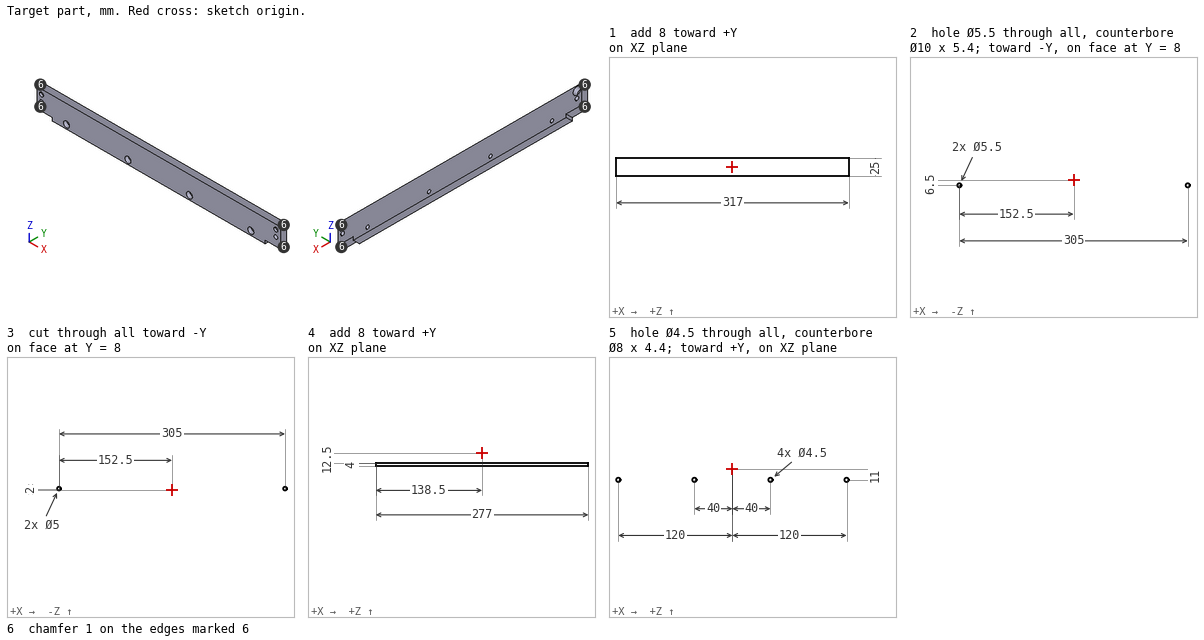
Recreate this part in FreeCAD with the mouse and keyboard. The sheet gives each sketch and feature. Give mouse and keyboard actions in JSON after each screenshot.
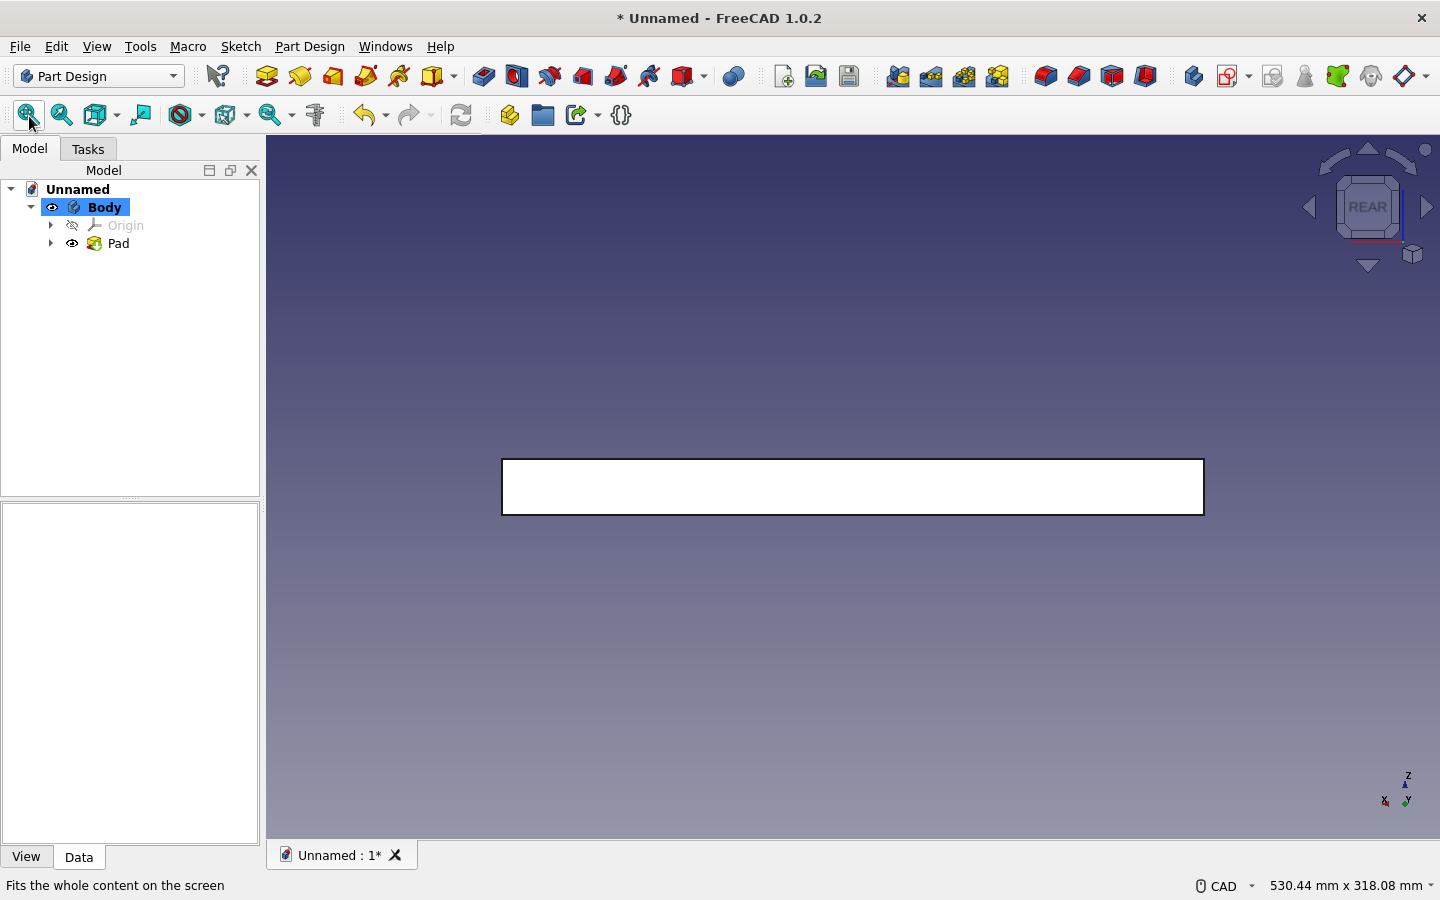
{"action": "left_click", "coordinate": [552, 486]}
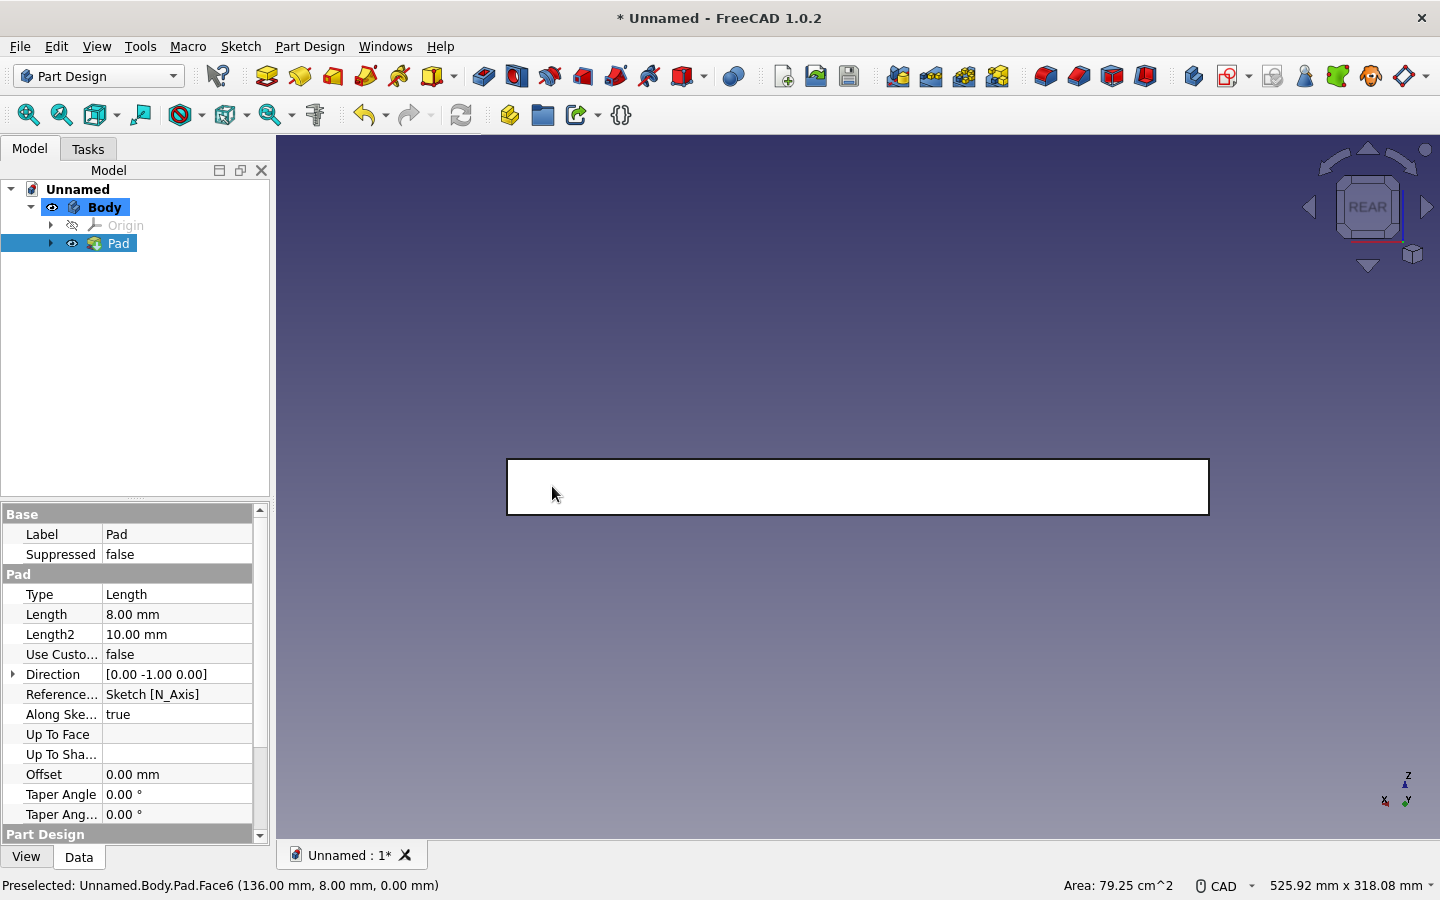
{"action": "left_click", "coordinate": [1226, 76]}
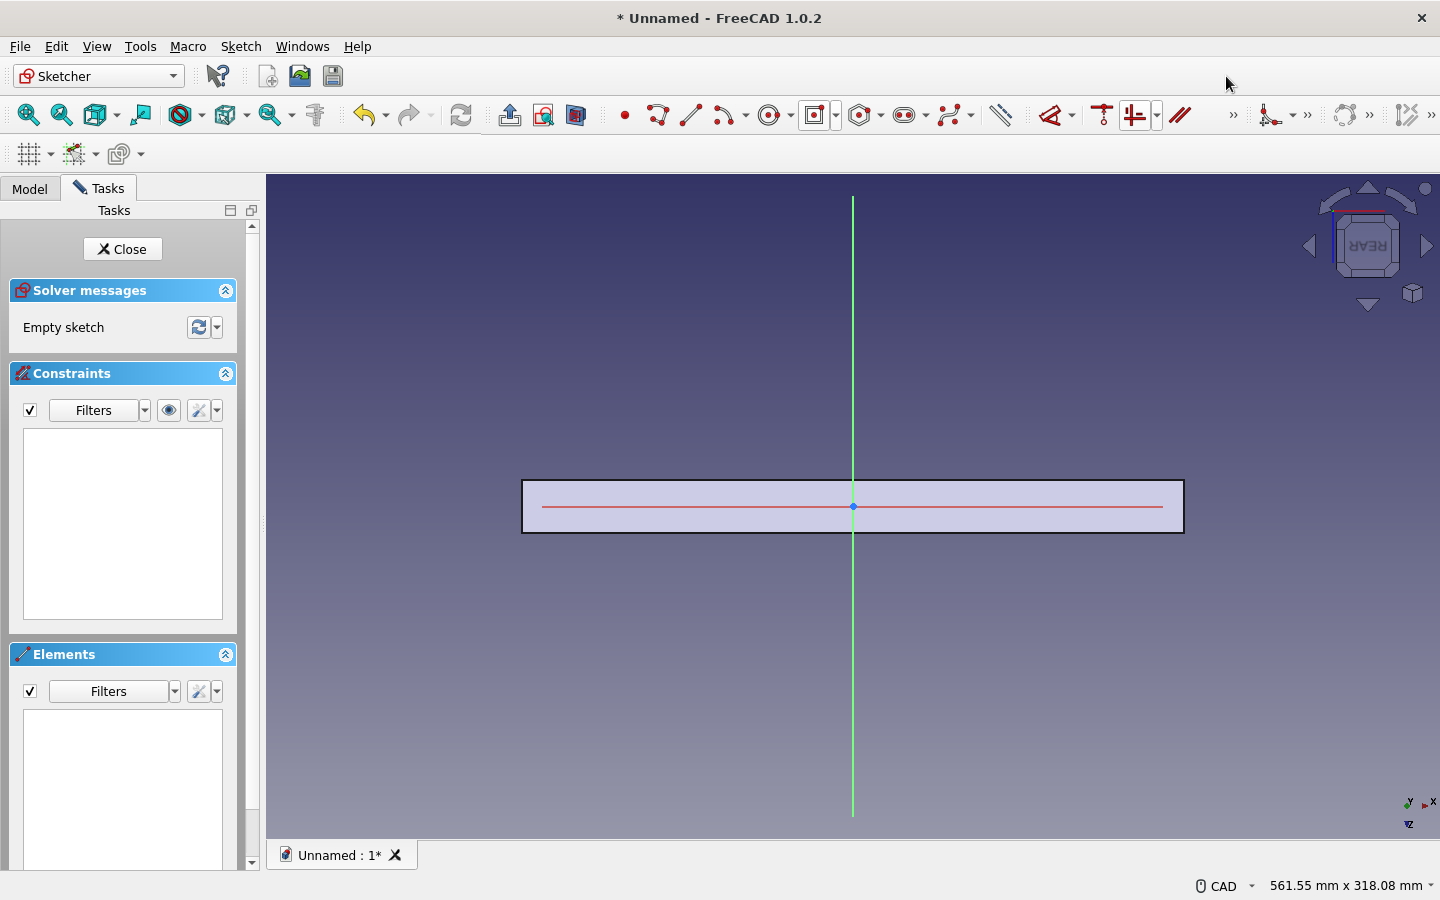
{"action": "left_click", "coordinate": [768, 116]}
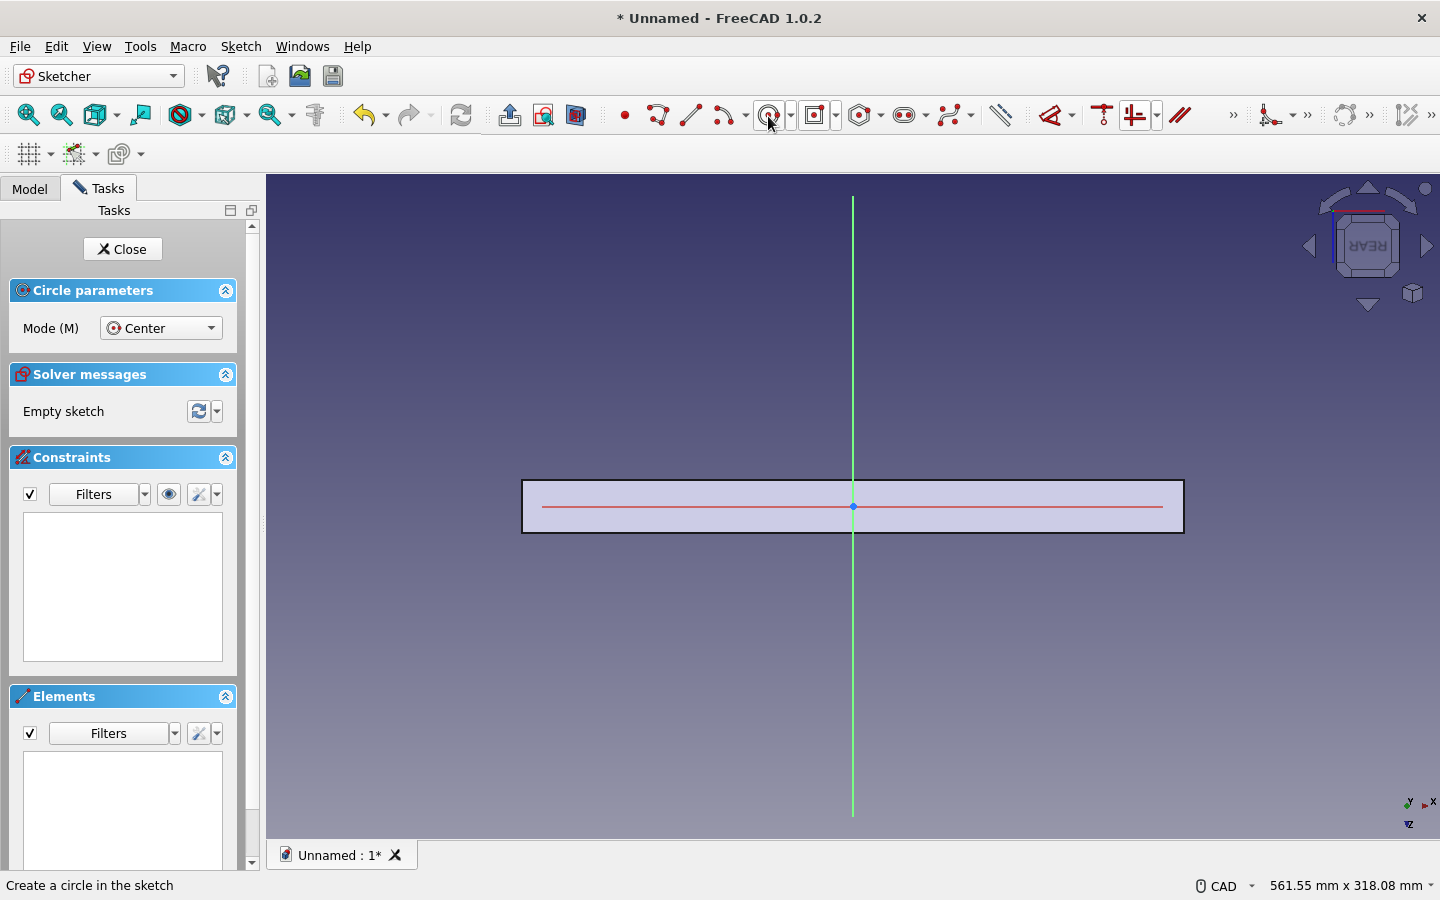
{"action": "scroll", "coordinate": [534, 520], "scroll_direction": "up", "scroll_amount": 7}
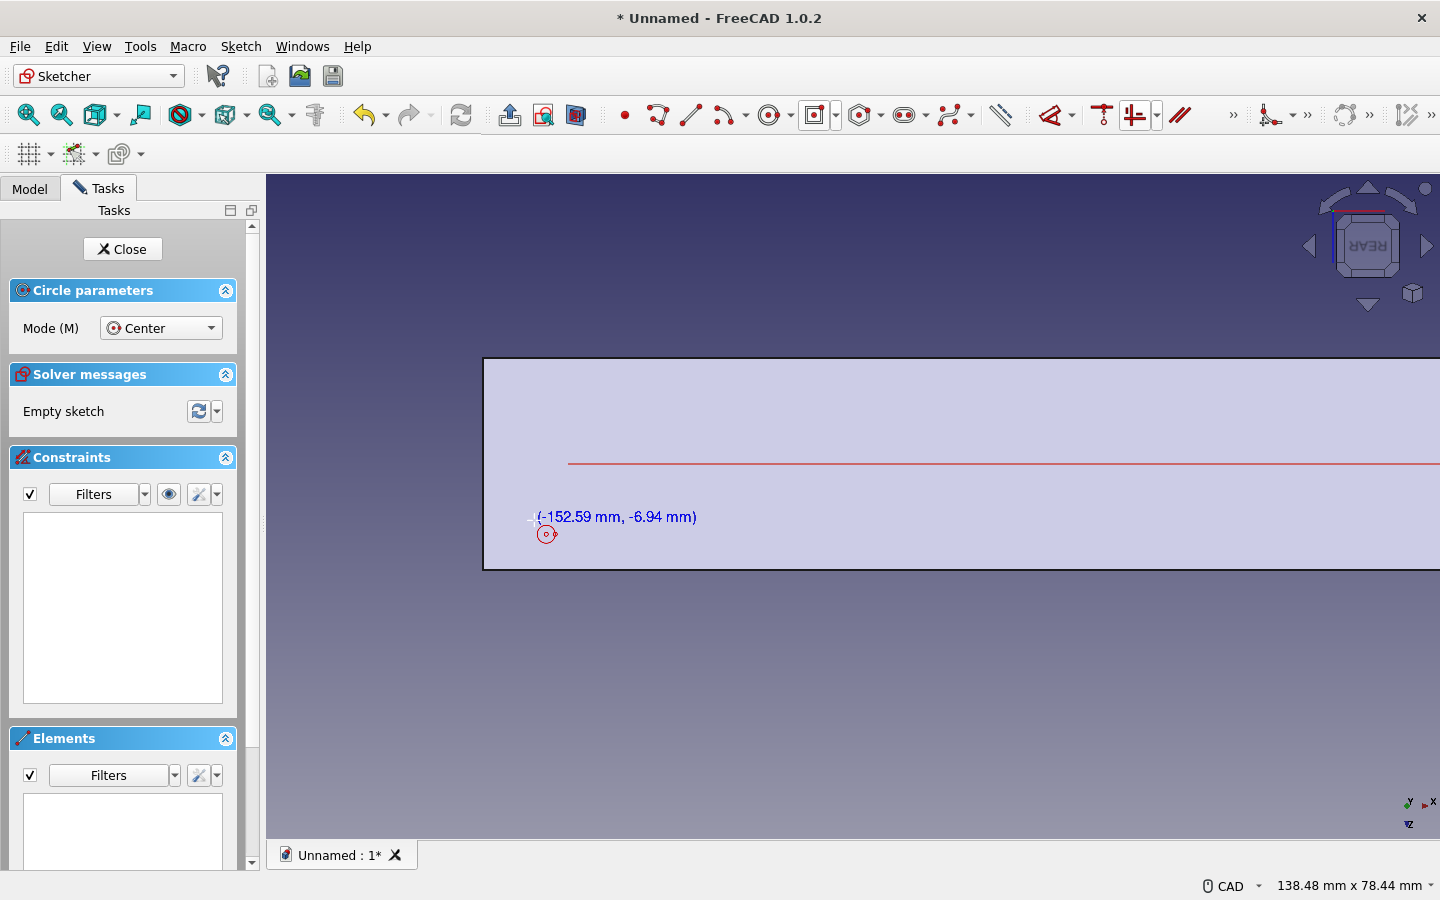
{"action": "scroll", "coordinate": [443, 508], "scroll_direction": "down", "scroll_amount": 7}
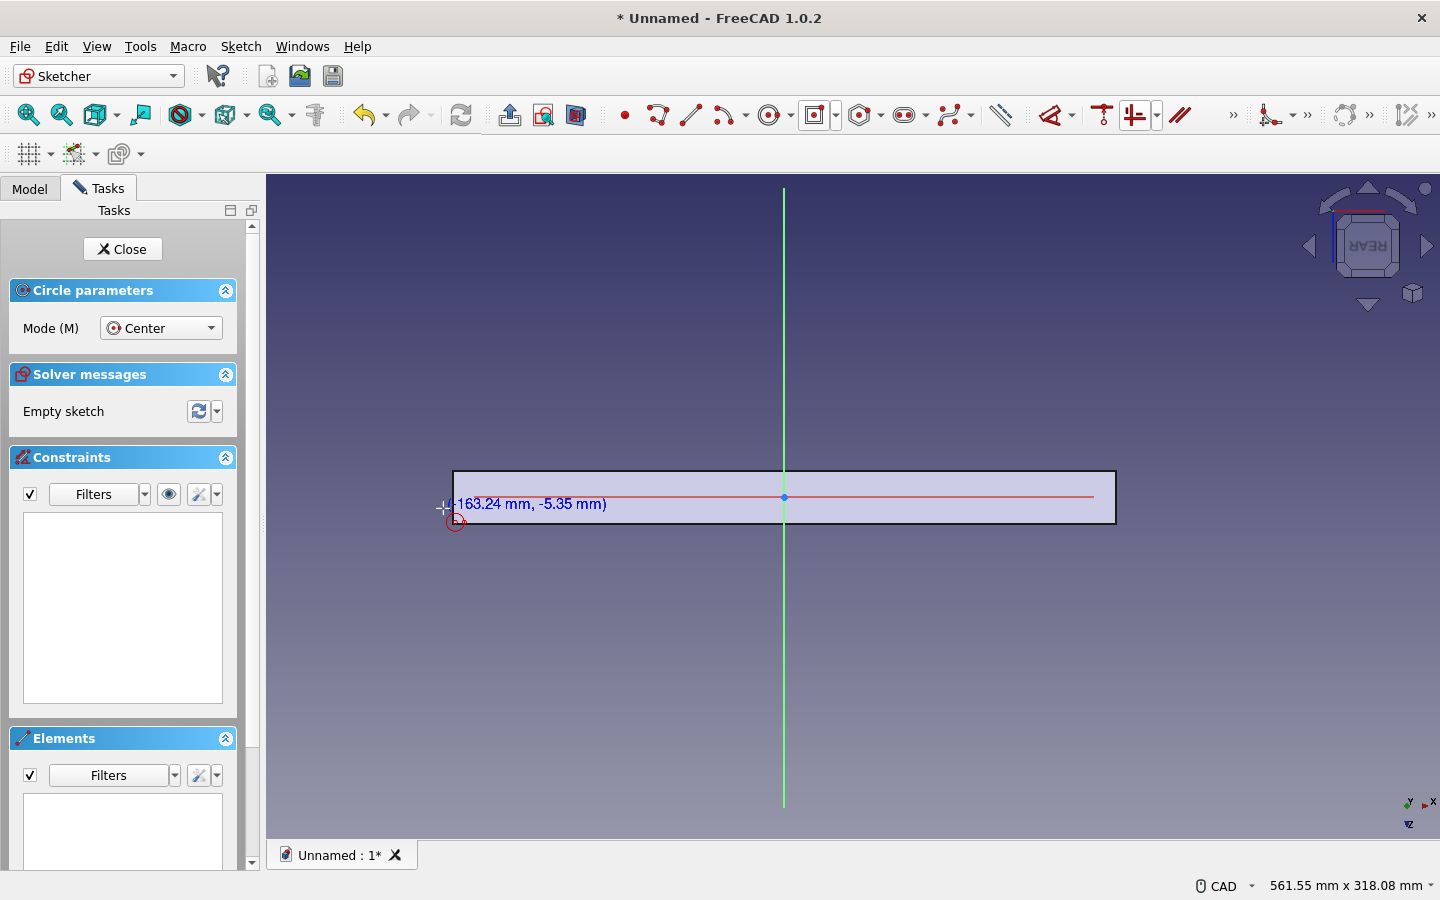
{"action": "left_click", "coordinate": [466, 511]}
{"action": "mouse_move", "coordinate": [470, 515]}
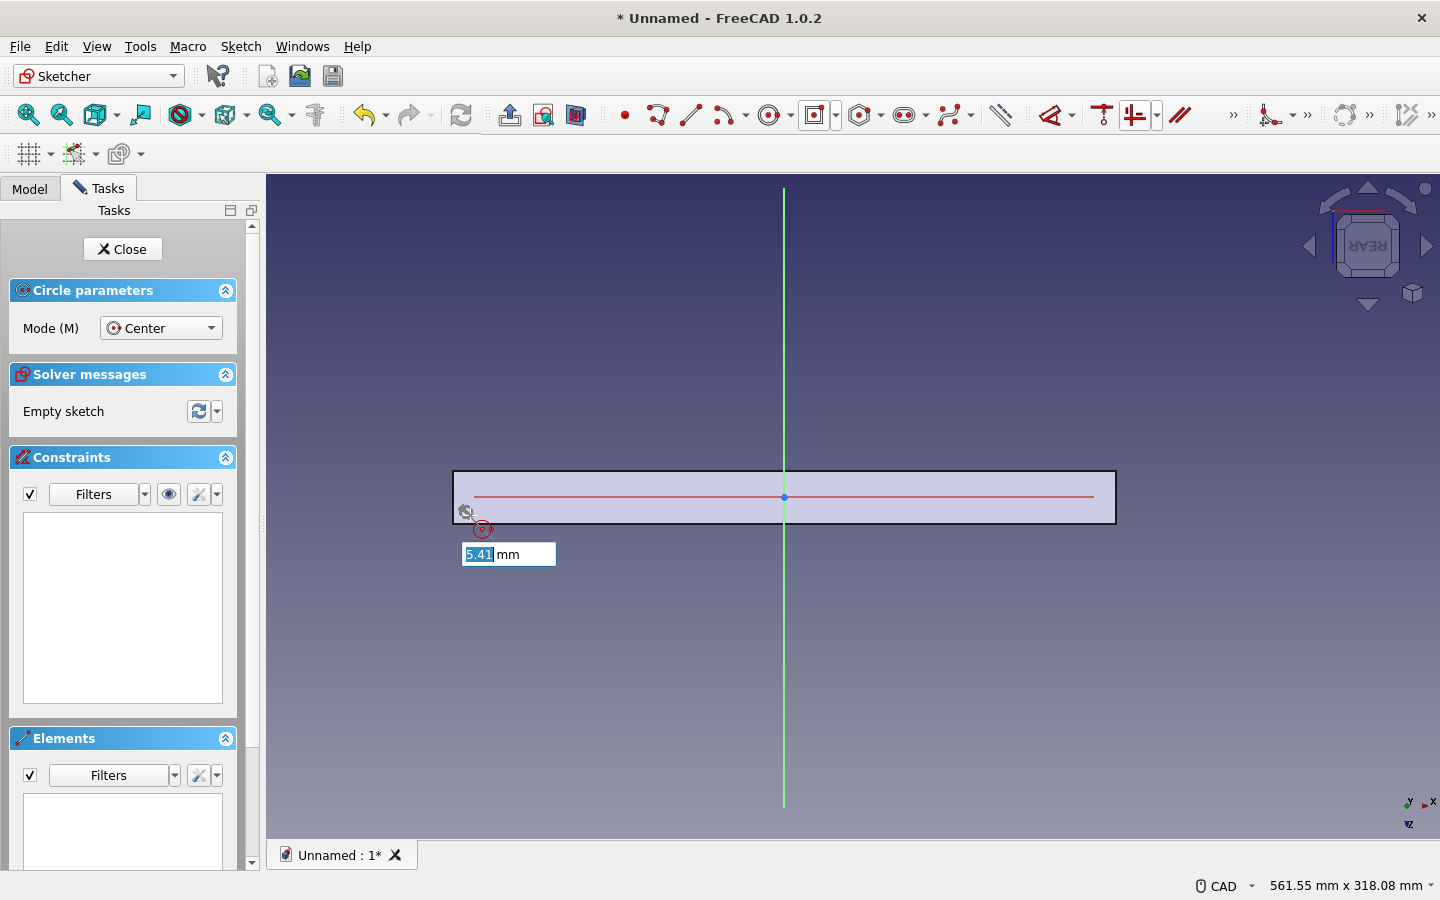
{"action": "type", "text": "5.5"}
{"action": "key", "text": "Return"}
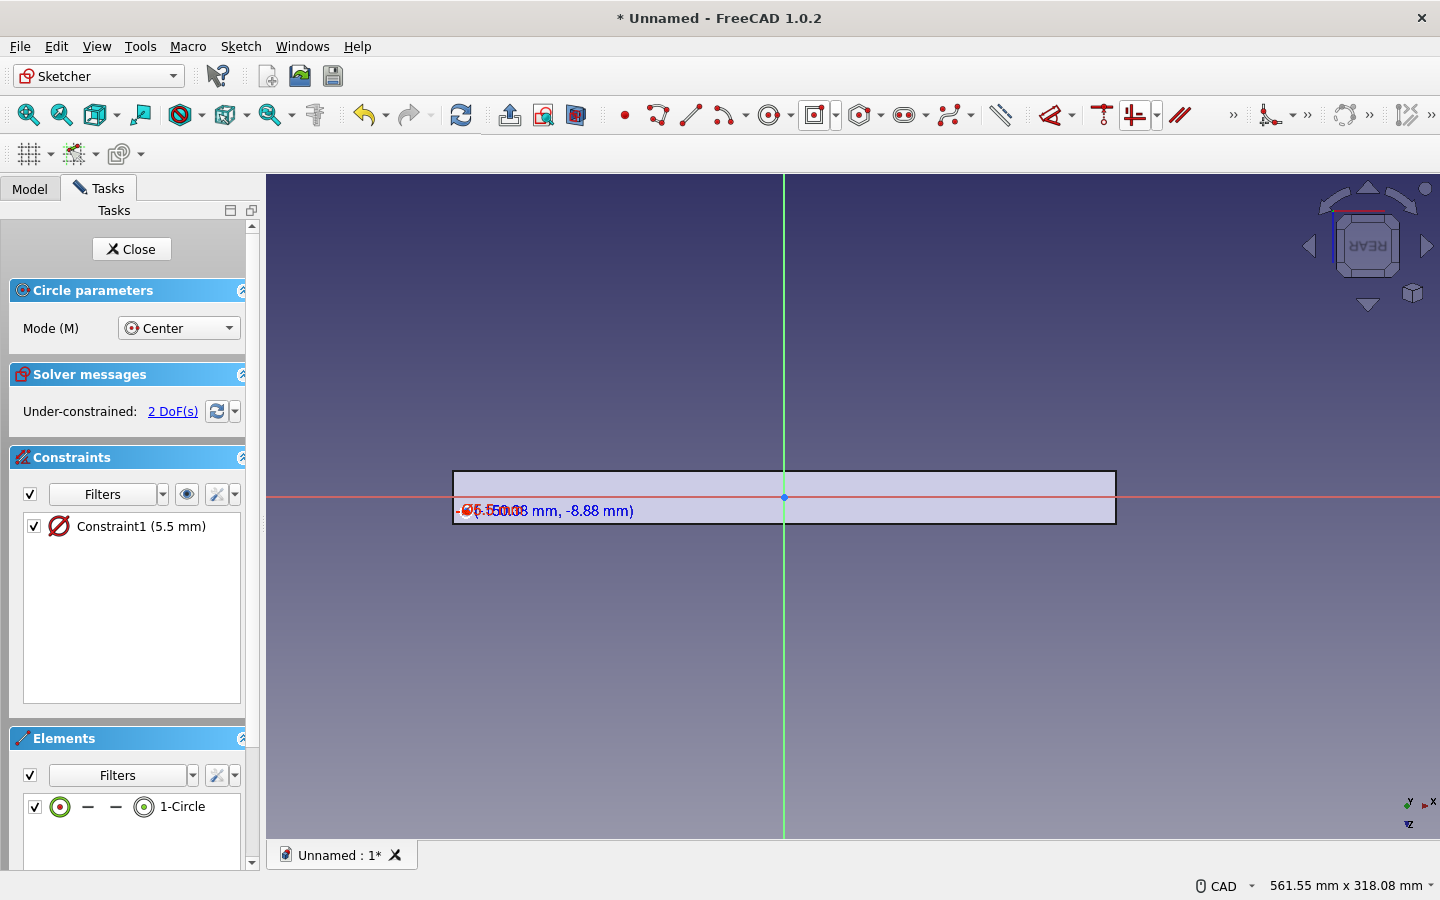
{"action": "scroll", "coordinate": [1103, 511], "scroll_direction": "up", "scroll_amount": 7}